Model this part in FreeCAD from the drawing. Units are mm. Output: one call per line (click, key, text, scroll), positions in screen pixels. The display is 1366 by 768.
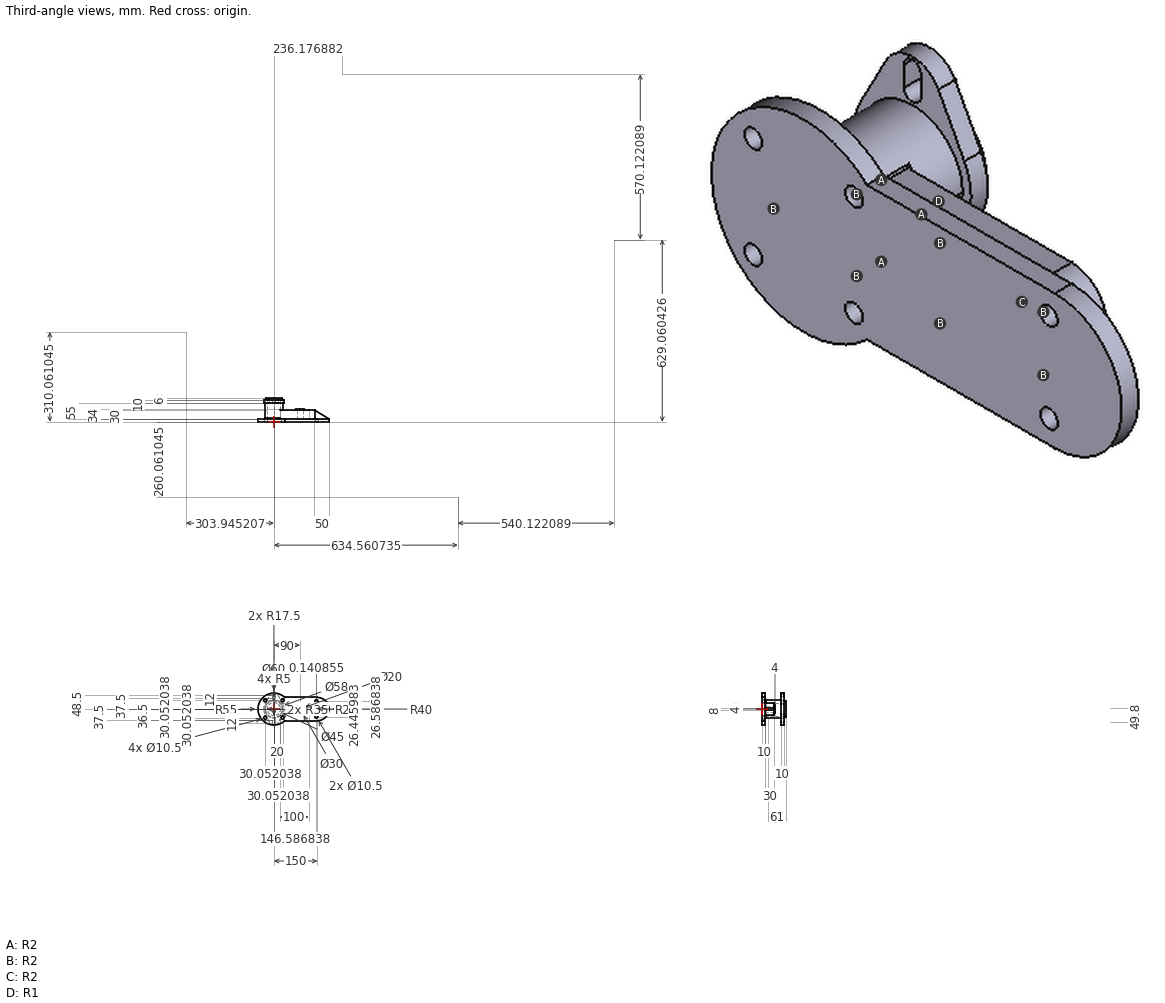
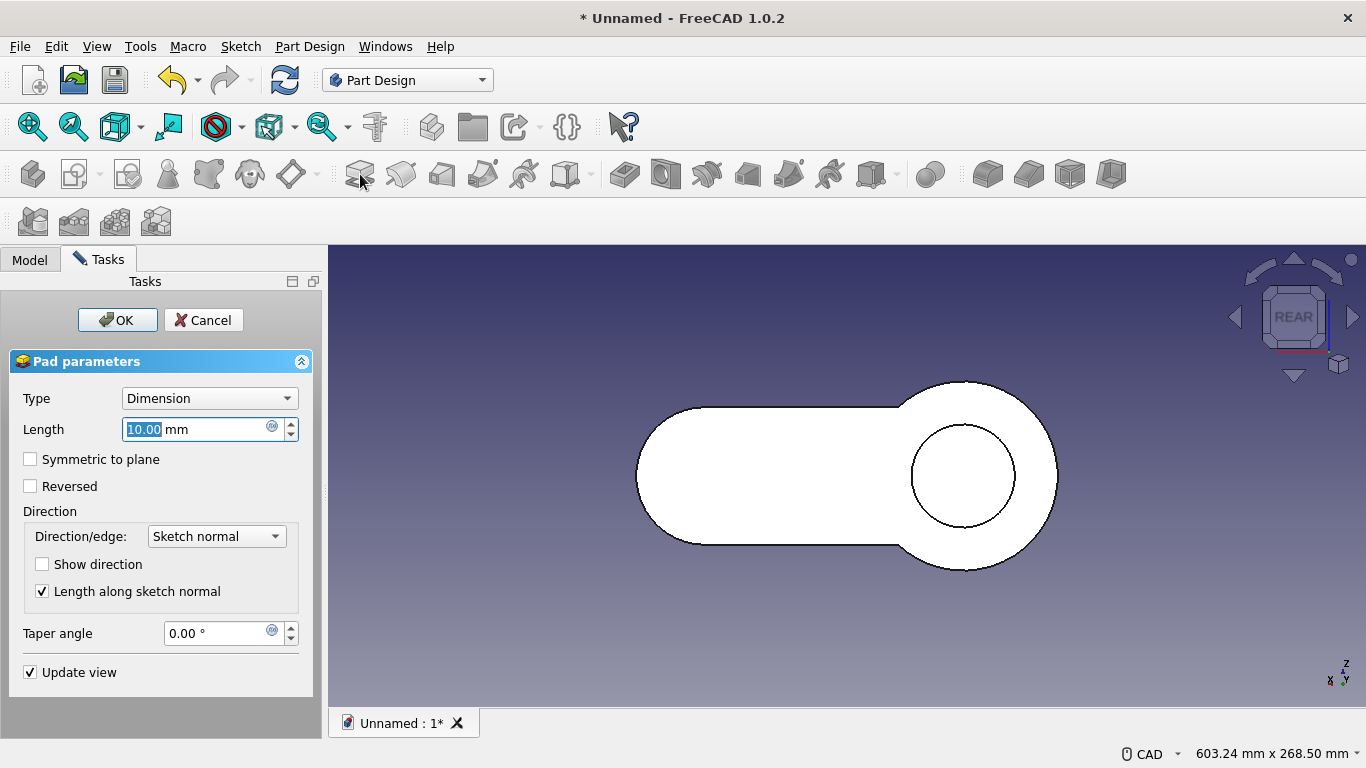
text(55)
key(Tab)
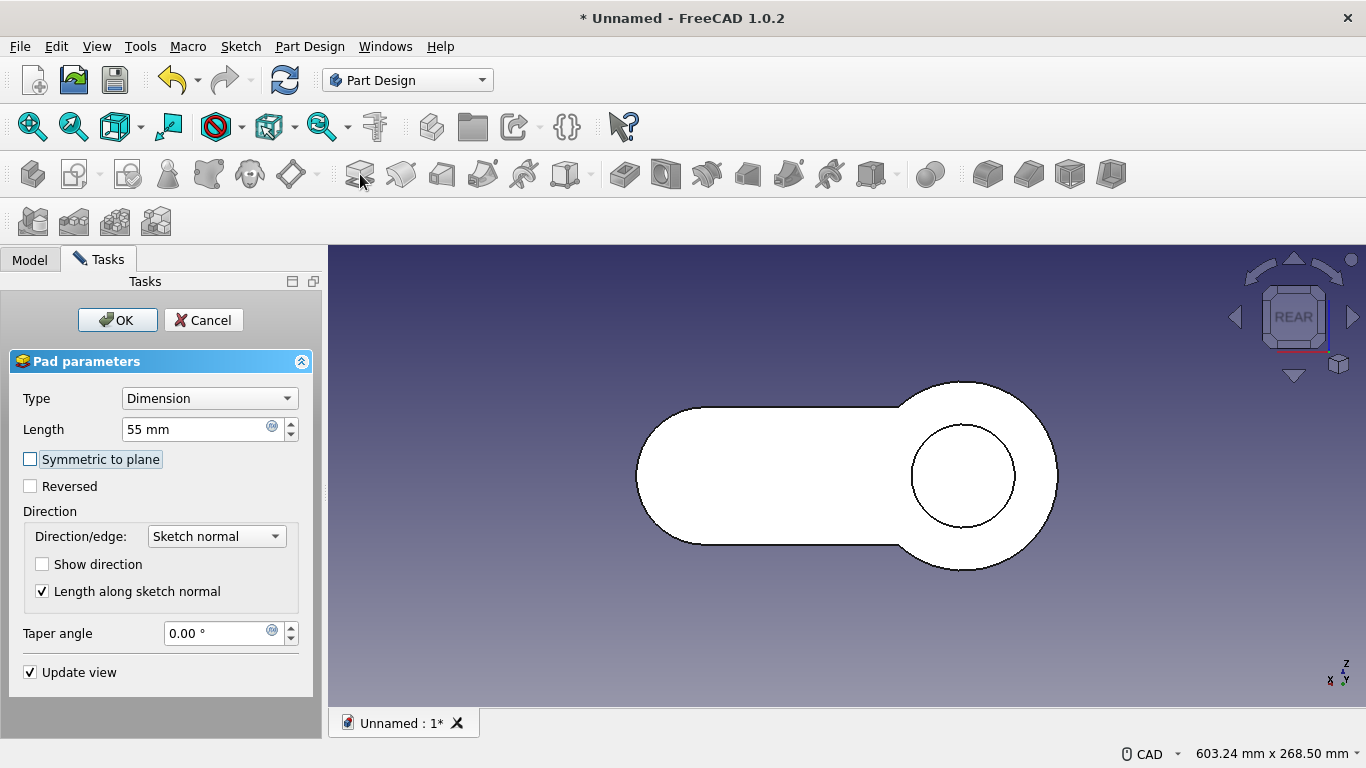
click(118, 320)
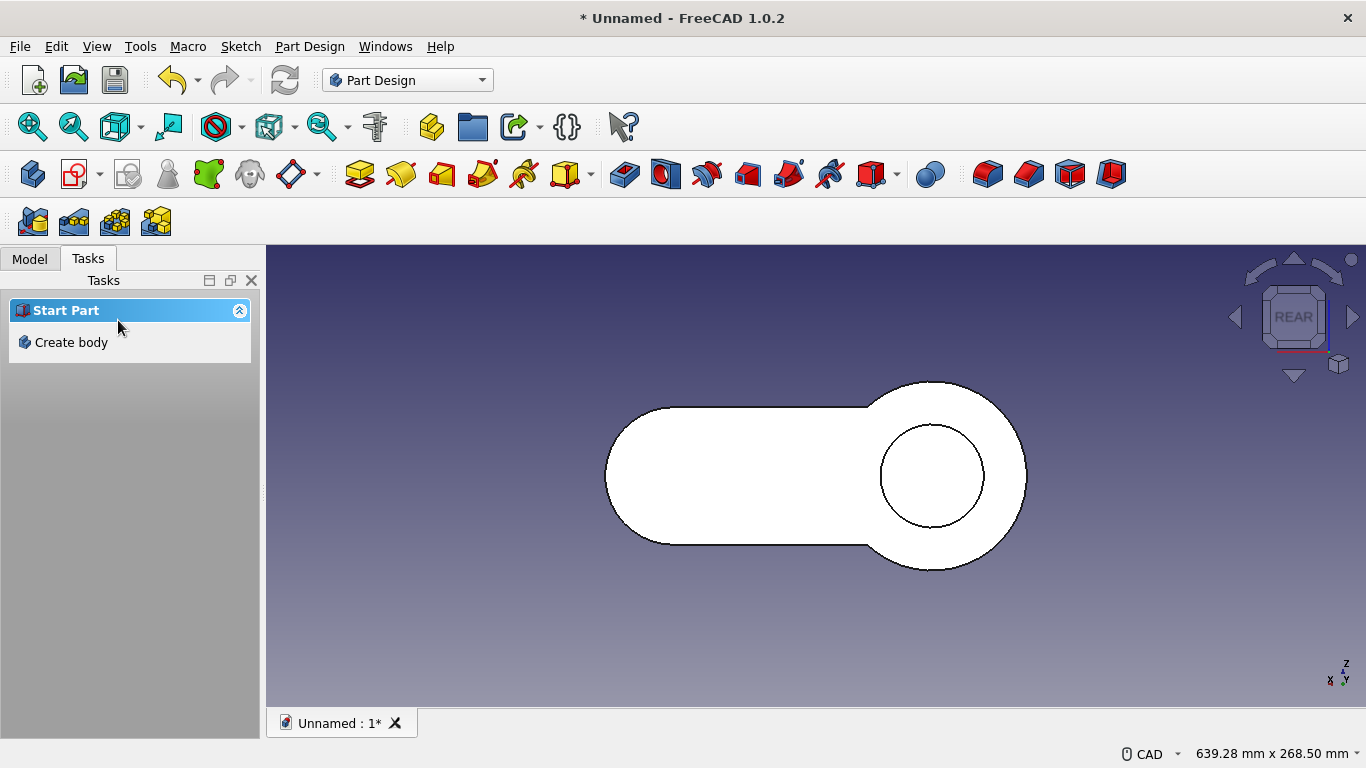
key(v)
key(f)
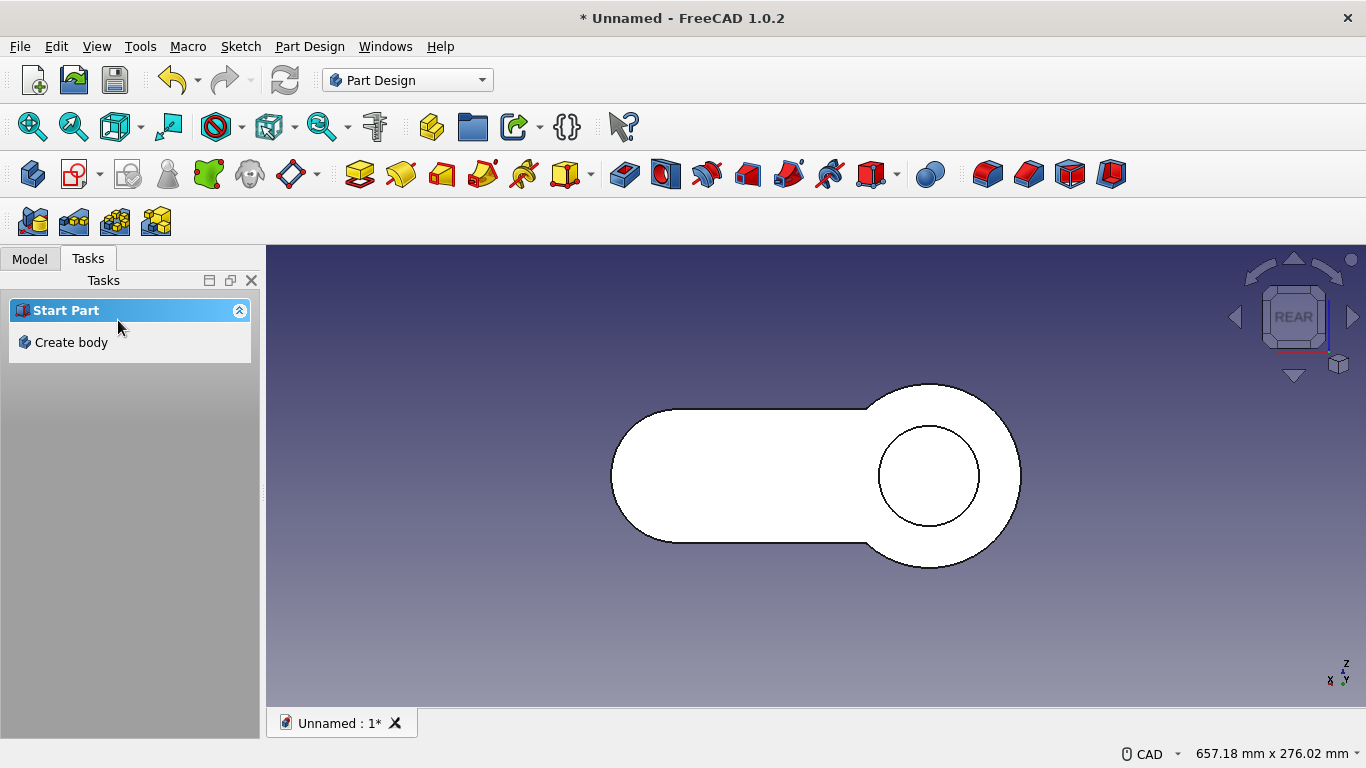
click(929, 475)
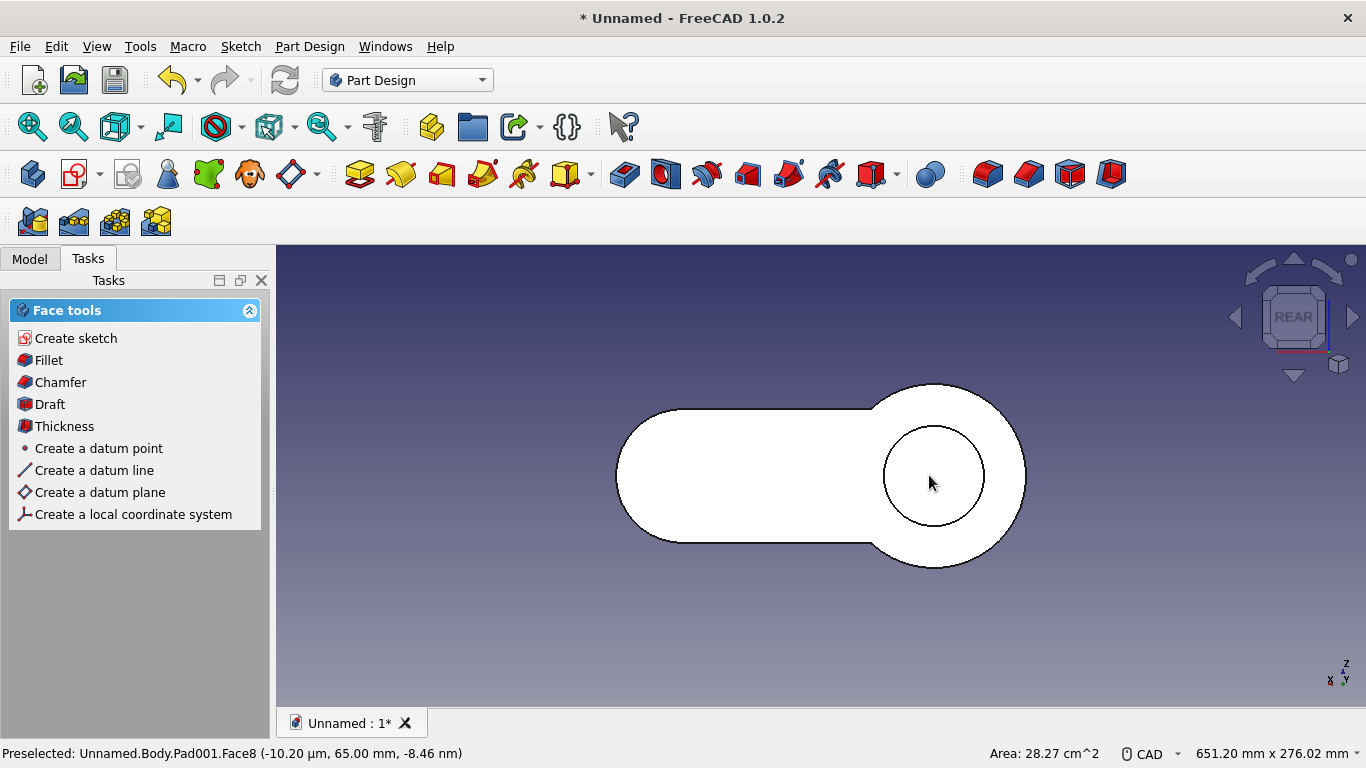
click(74, 174)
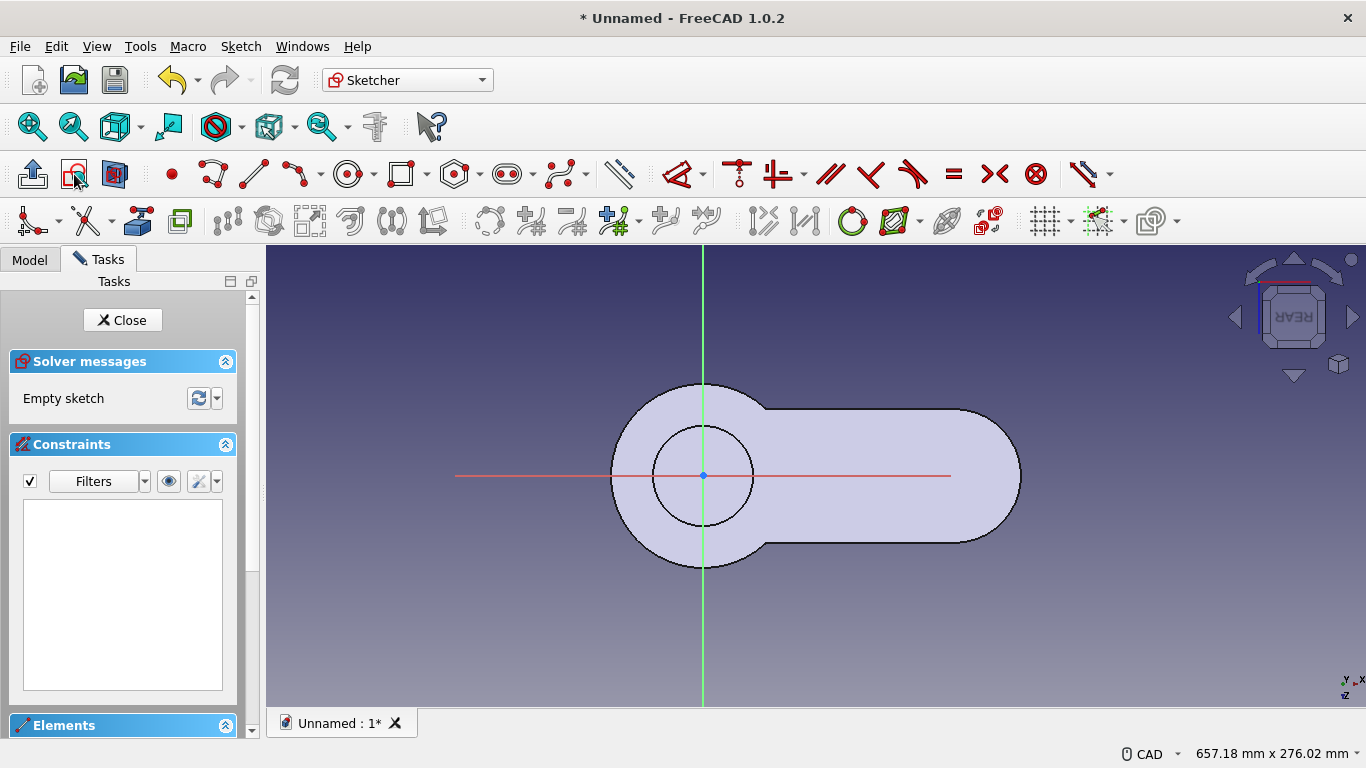
scroll(613, 476, up, 2)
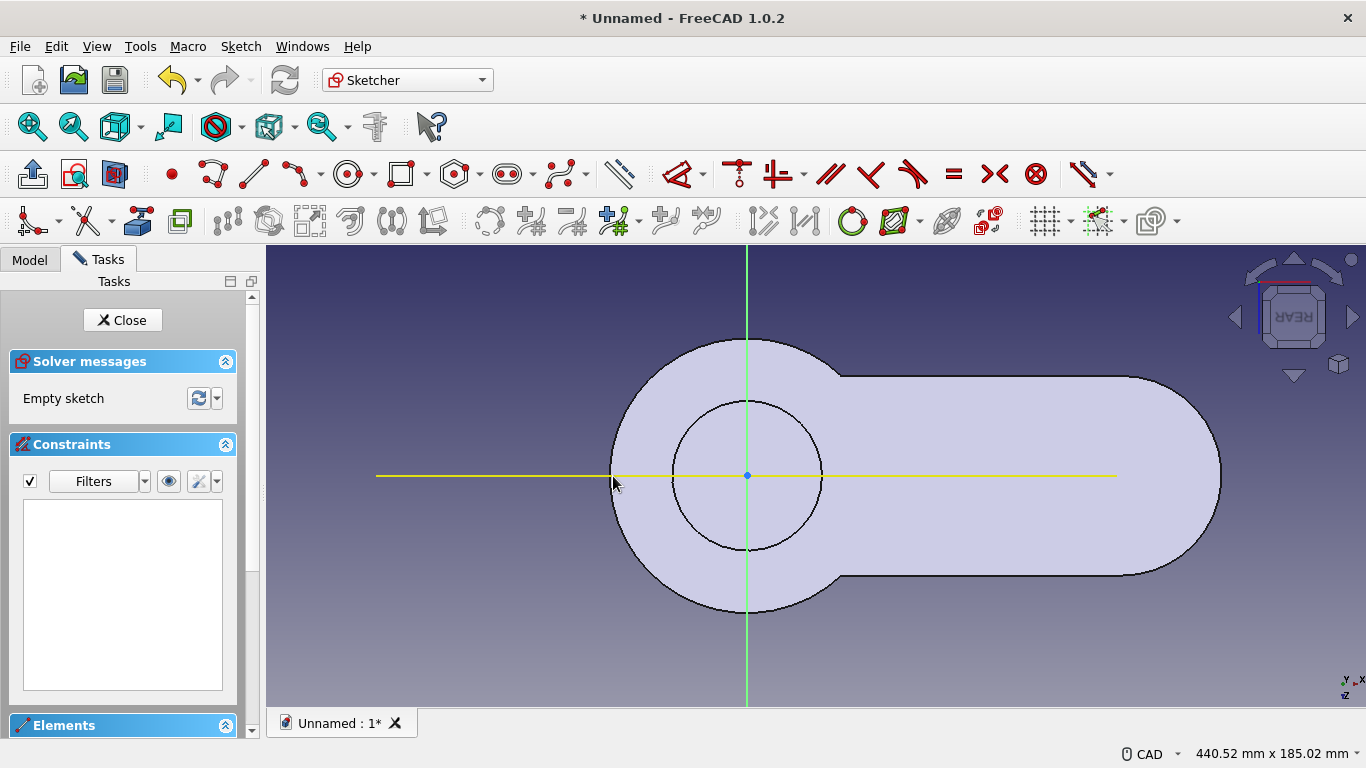
key(g)
key(l)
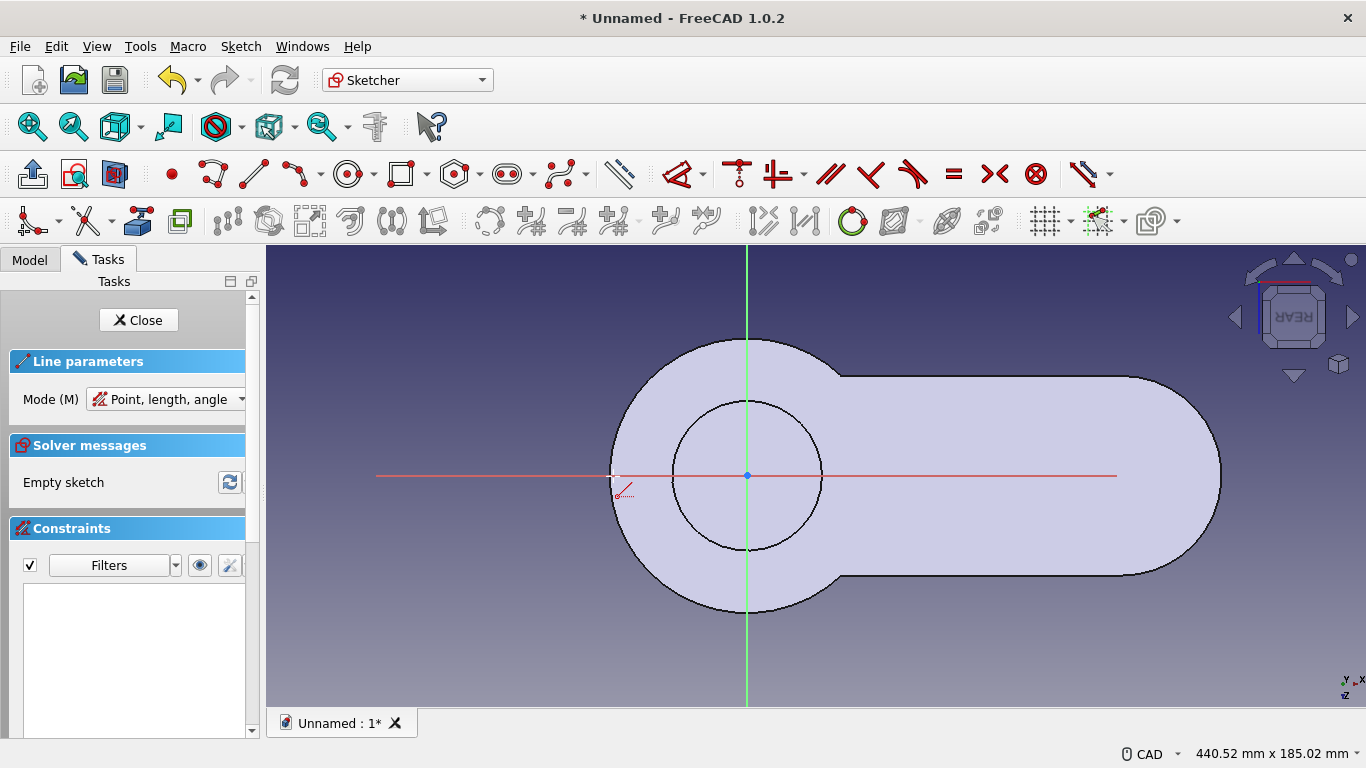
click(708, 362)
click(670, 435)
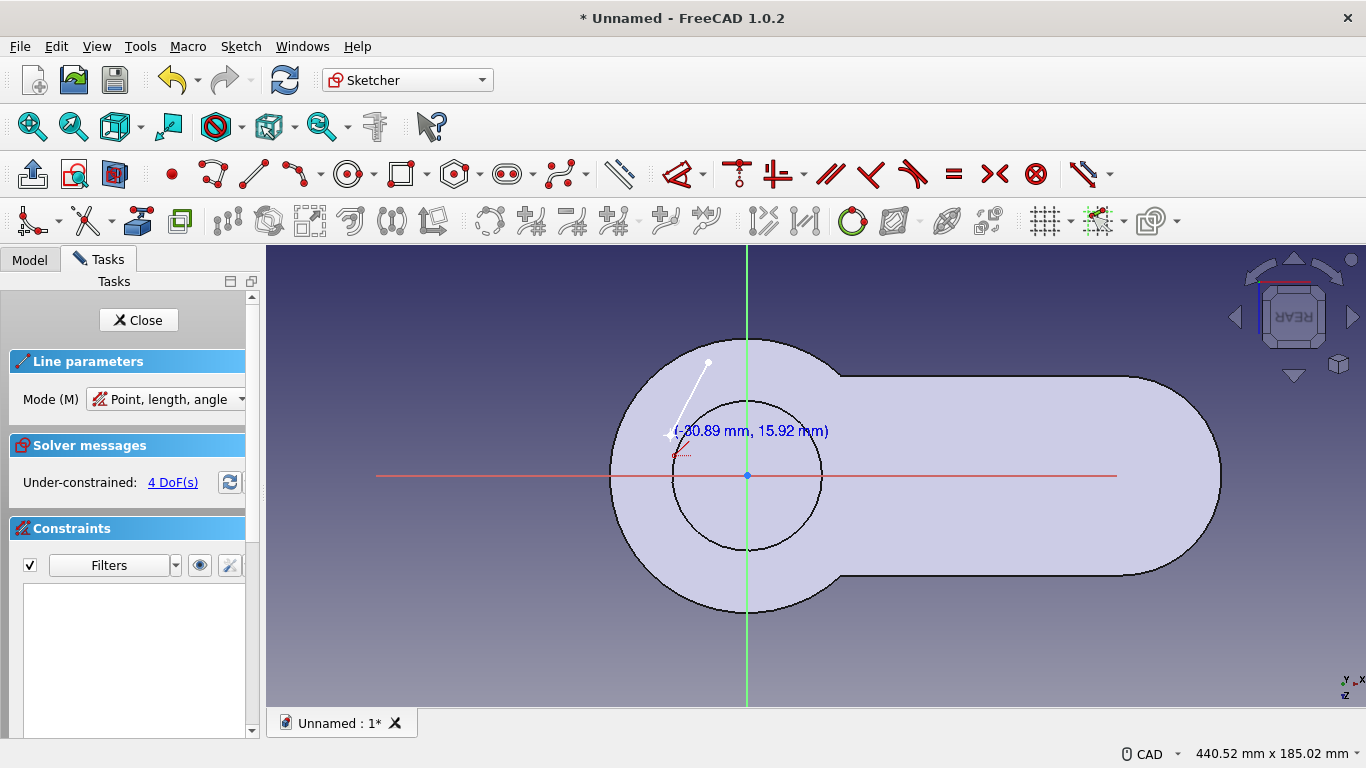
click(670, 517)
click(708, 590)